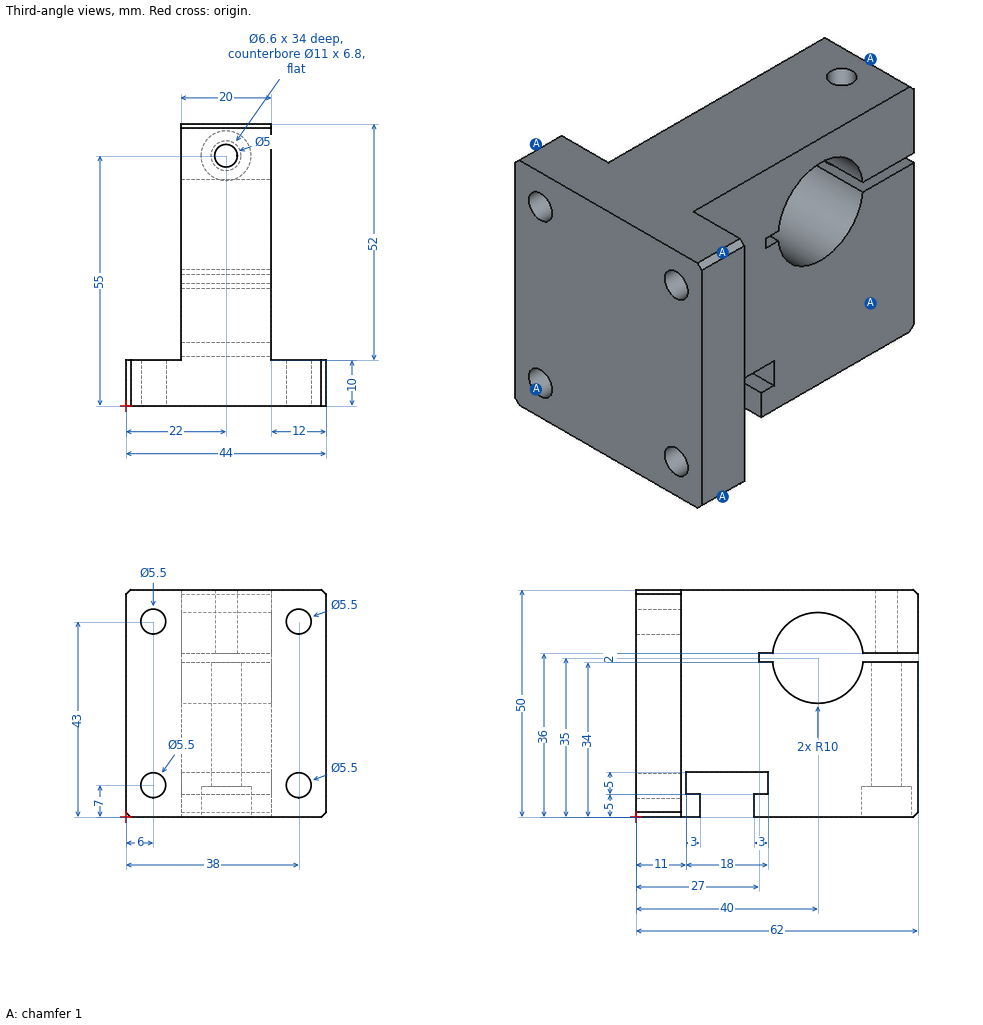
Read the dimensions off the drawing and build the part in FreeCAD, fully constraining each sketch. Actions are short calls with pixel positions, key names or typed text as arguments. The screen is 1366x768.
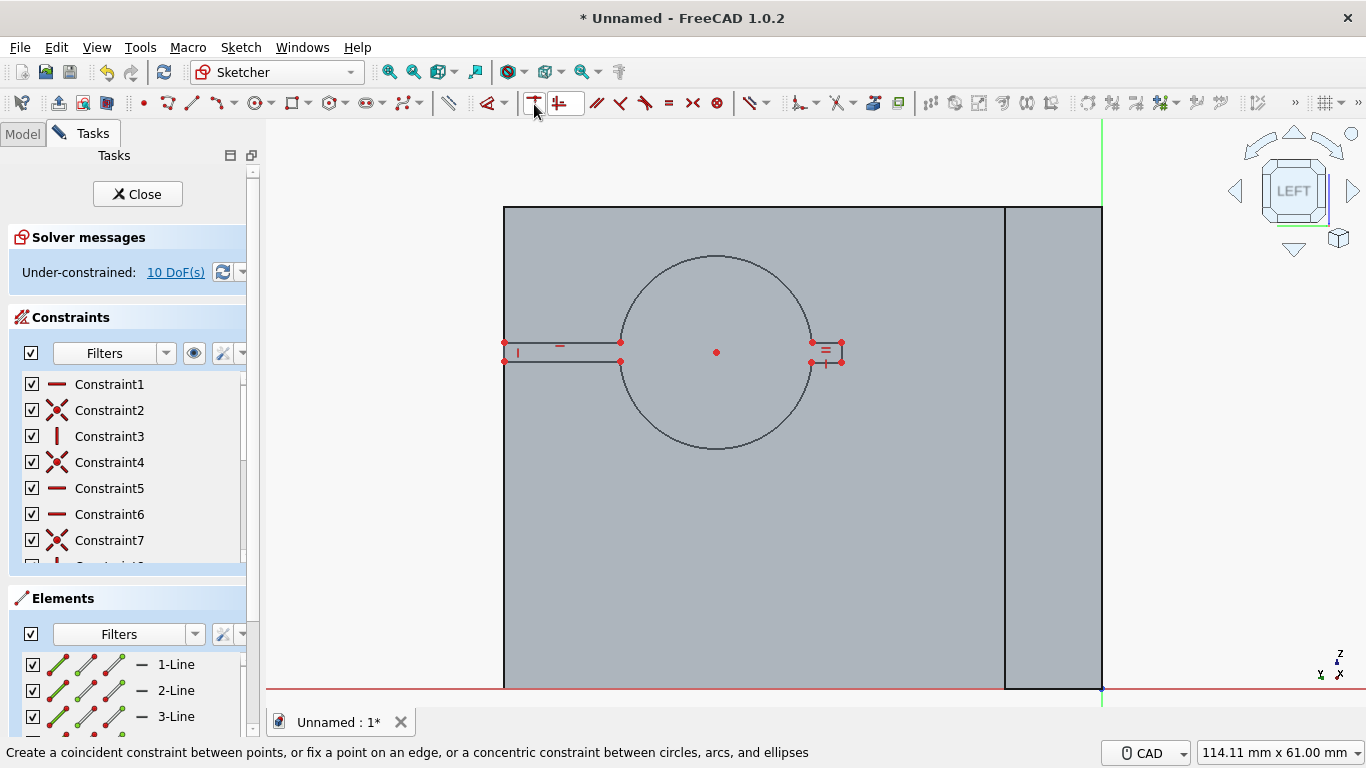
click(770, 272)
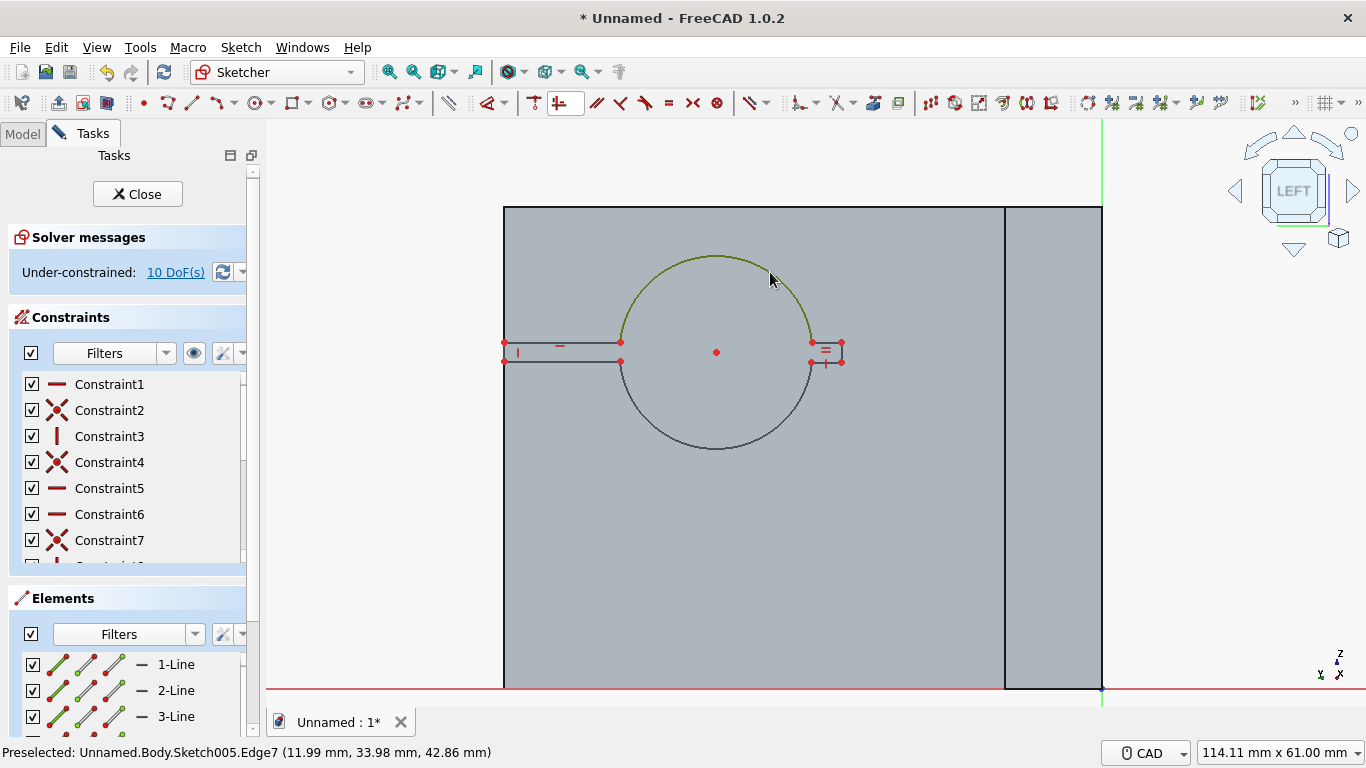
click(662, 433)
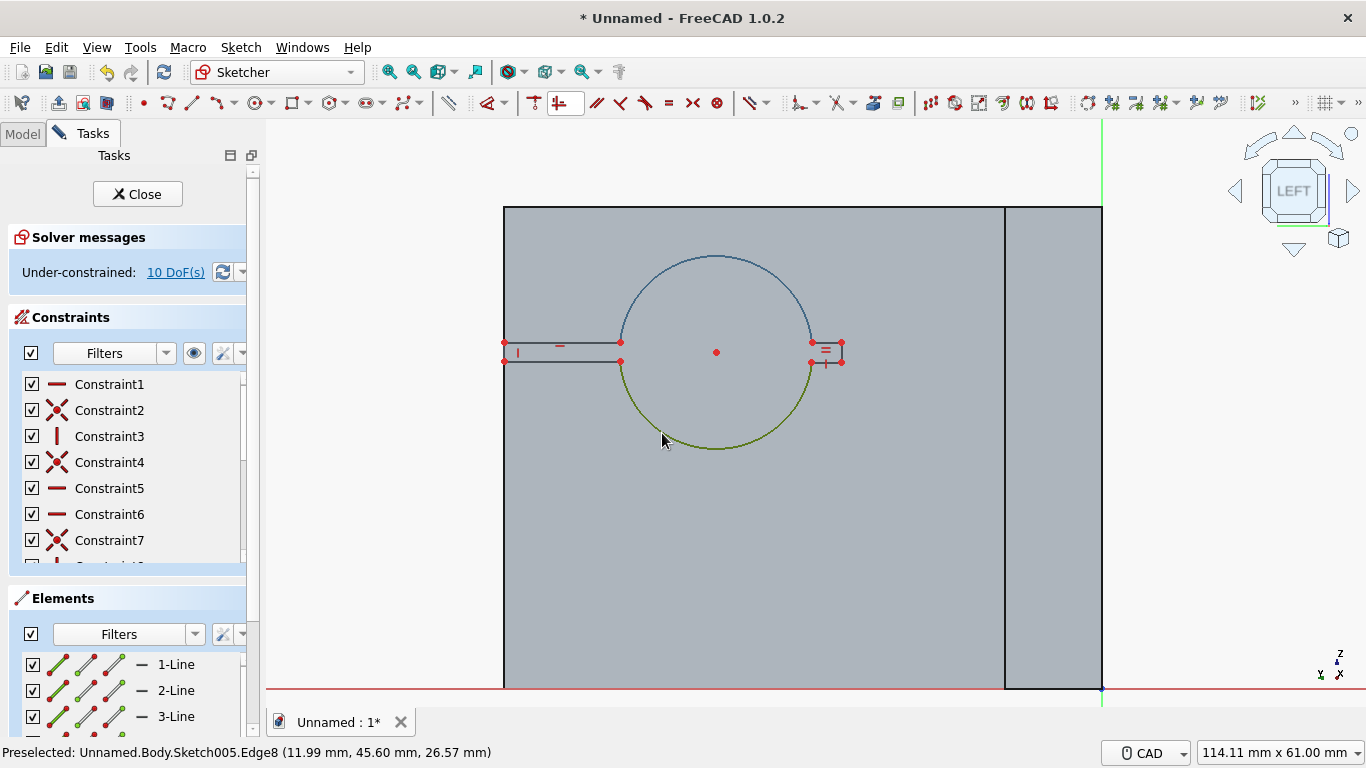
click(670, 104)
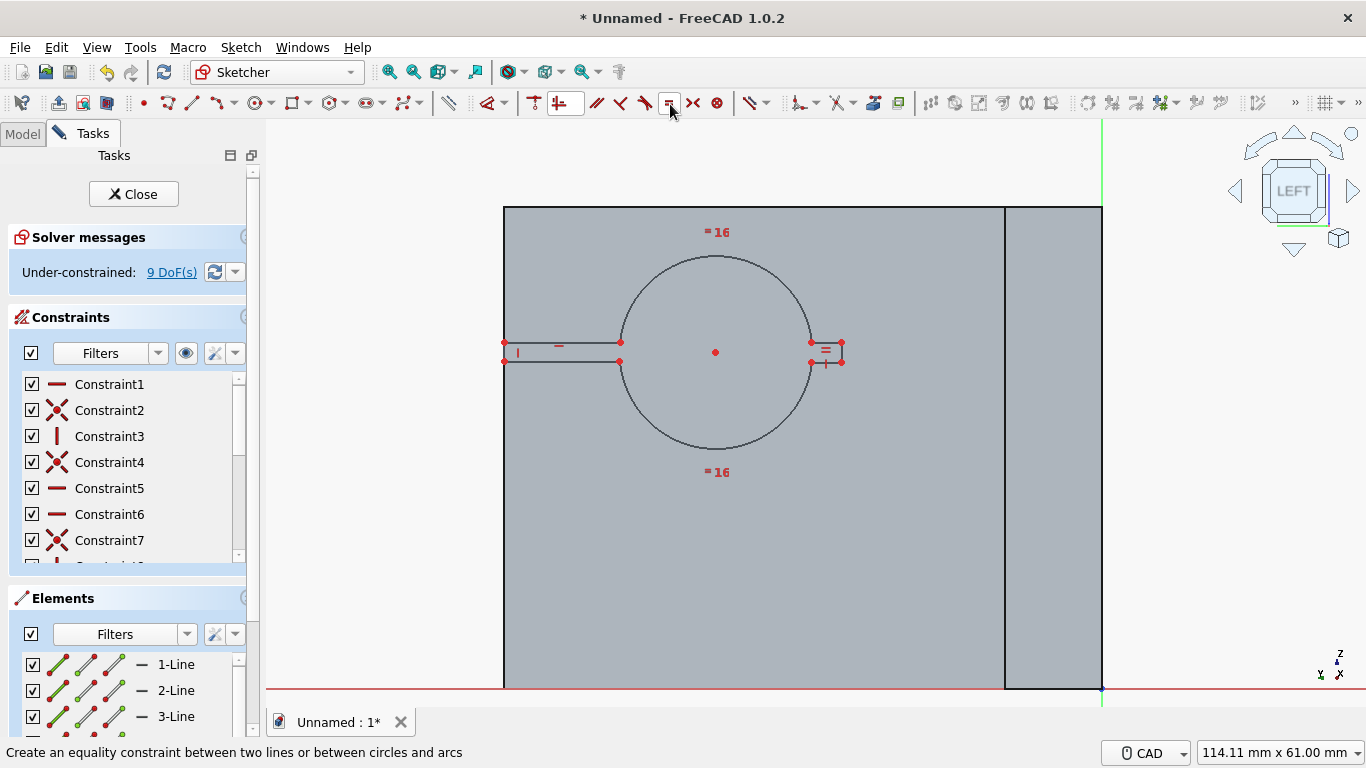
click(488, 104)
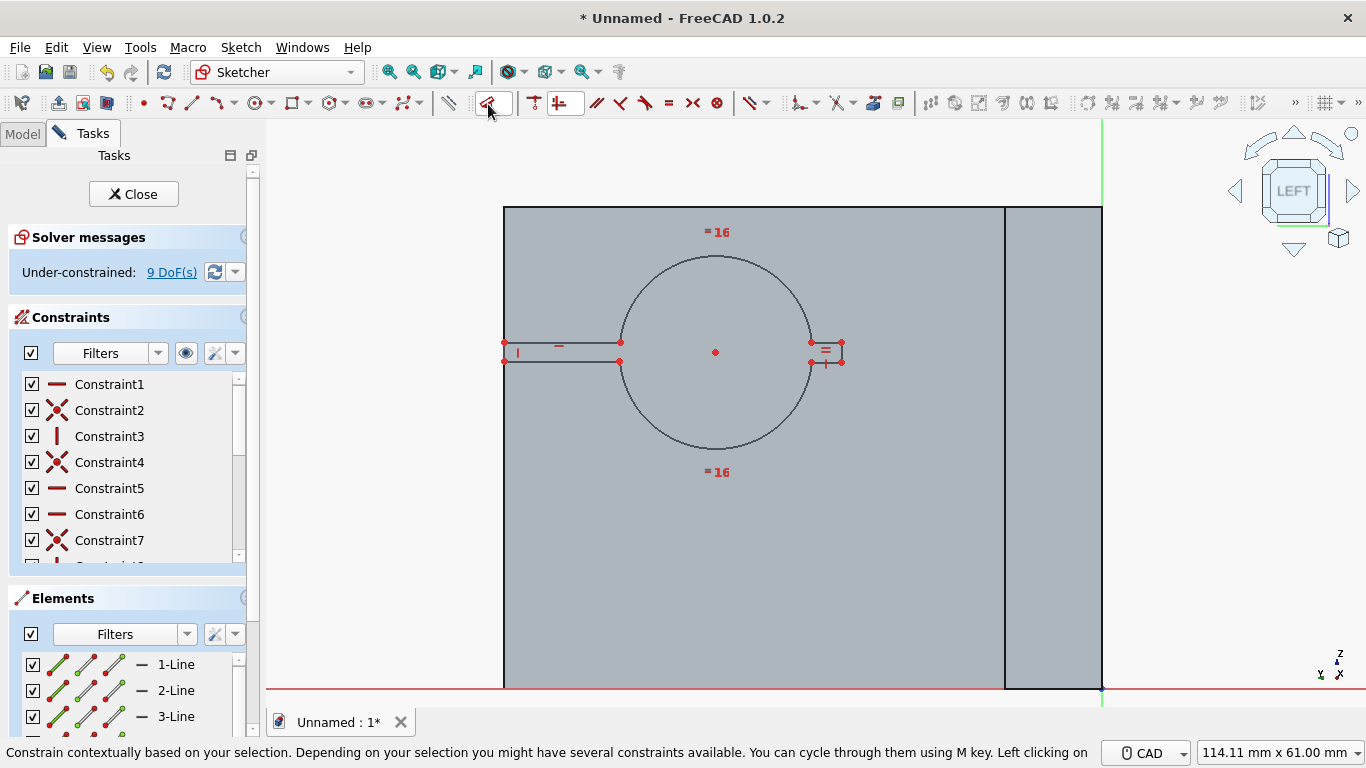
click(770, 272)
click(788, 245)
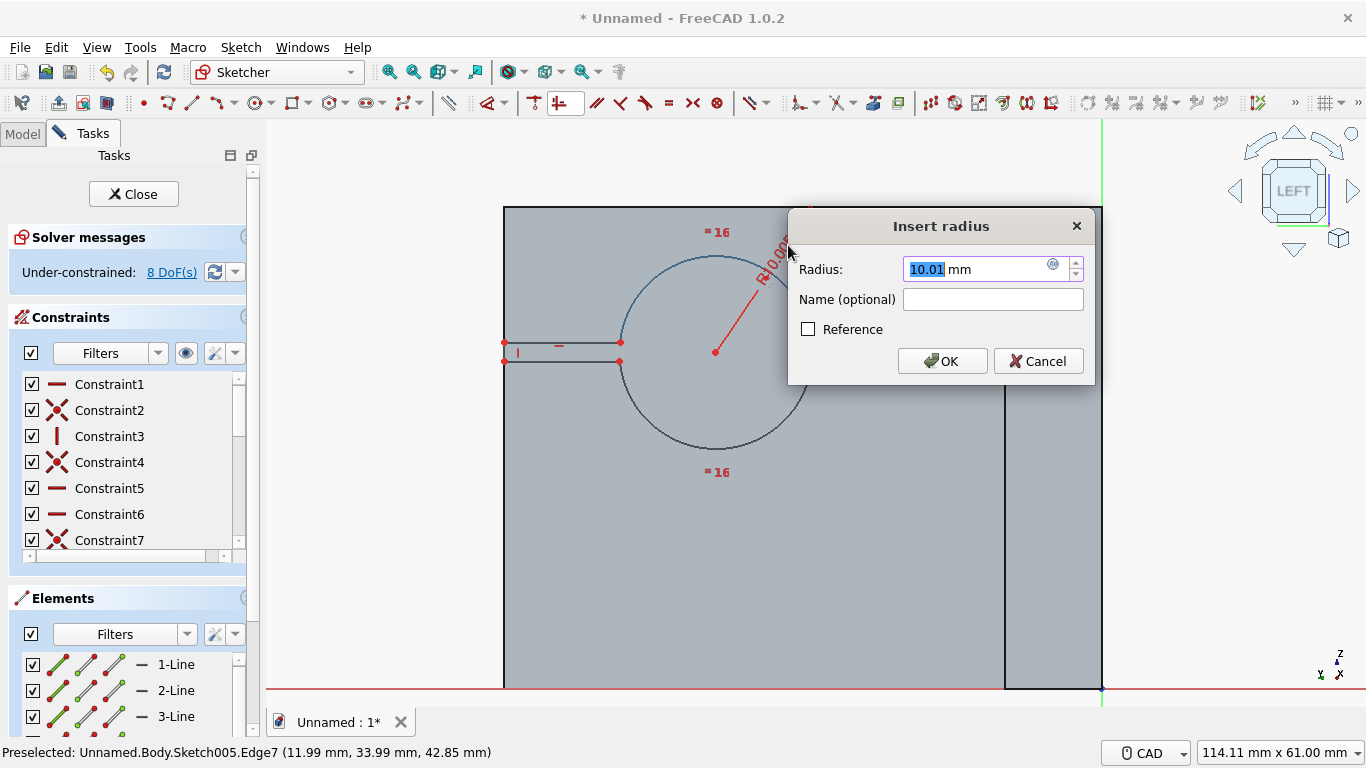
text(10)
key(Return)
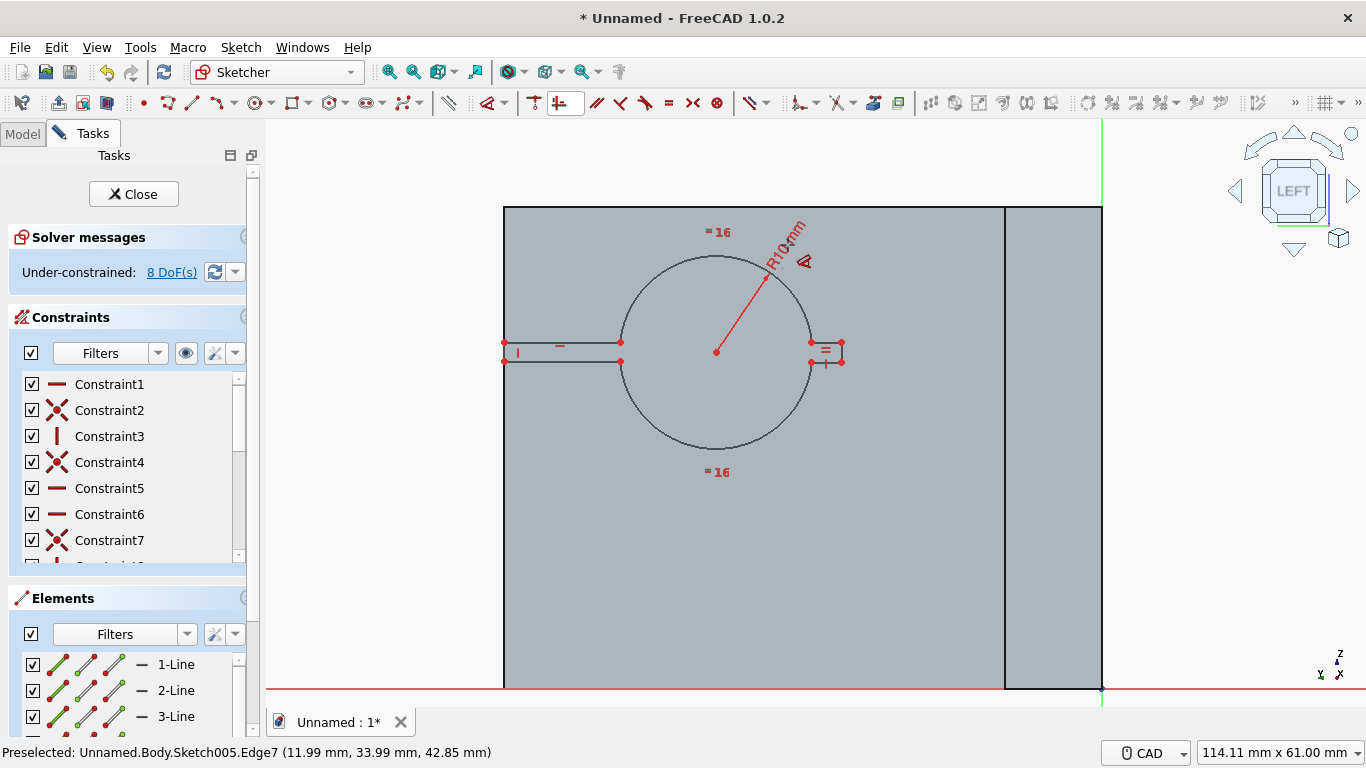
scroll(842, 353, up, 4)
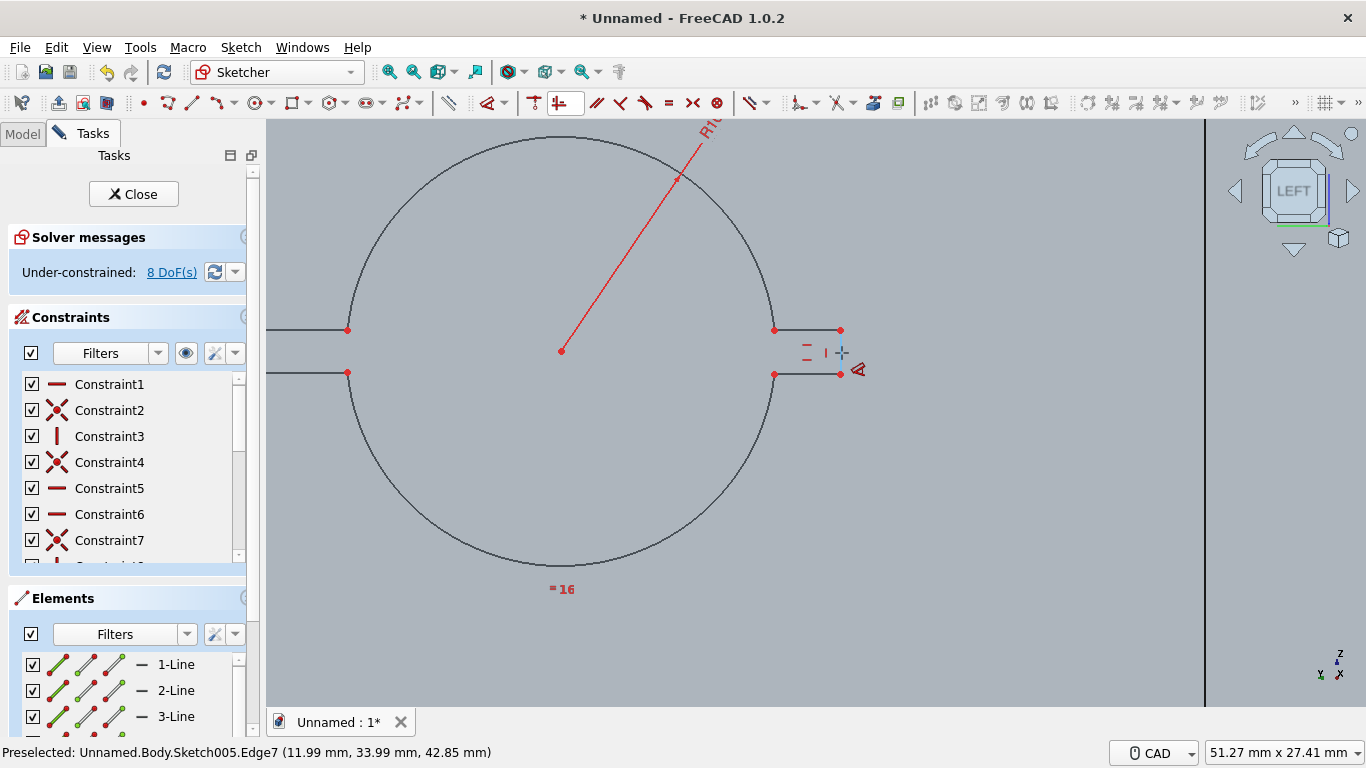
click(841, 352)
click(875, 352)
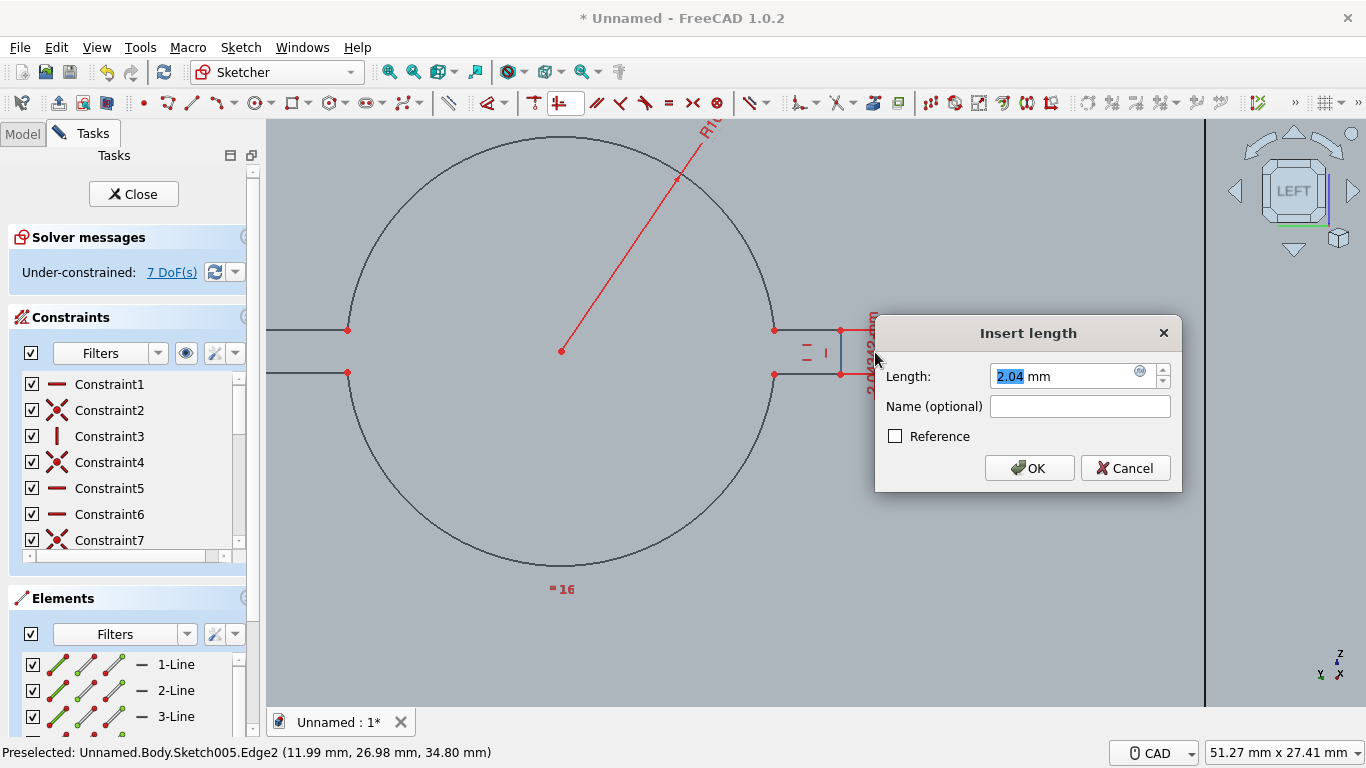
text(2)
key(Return)